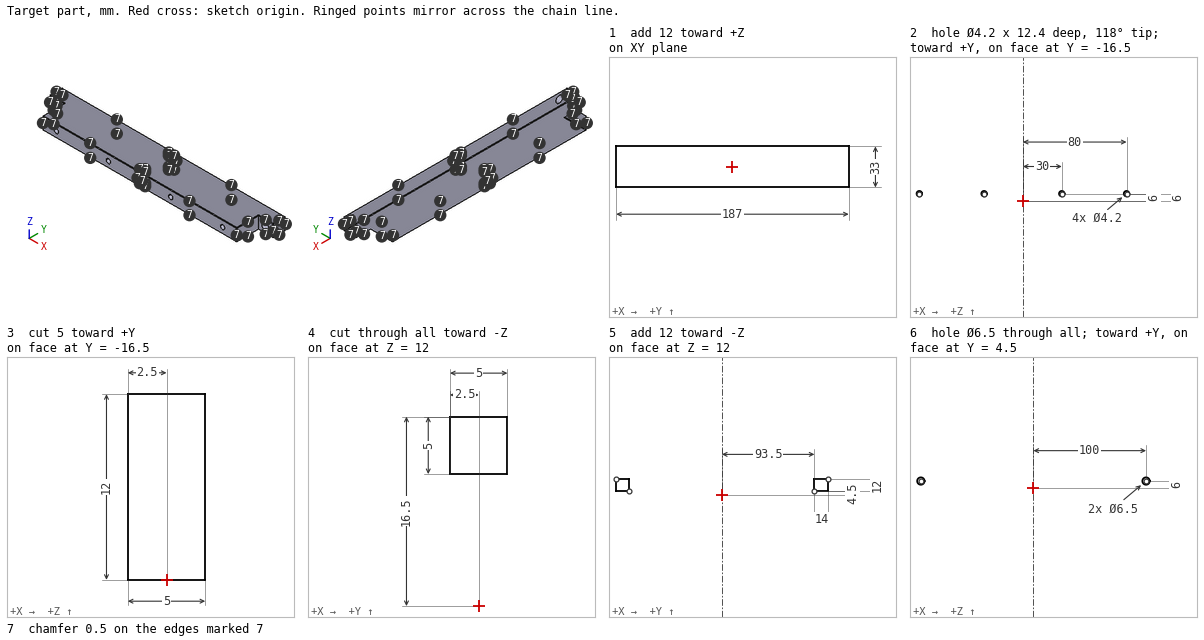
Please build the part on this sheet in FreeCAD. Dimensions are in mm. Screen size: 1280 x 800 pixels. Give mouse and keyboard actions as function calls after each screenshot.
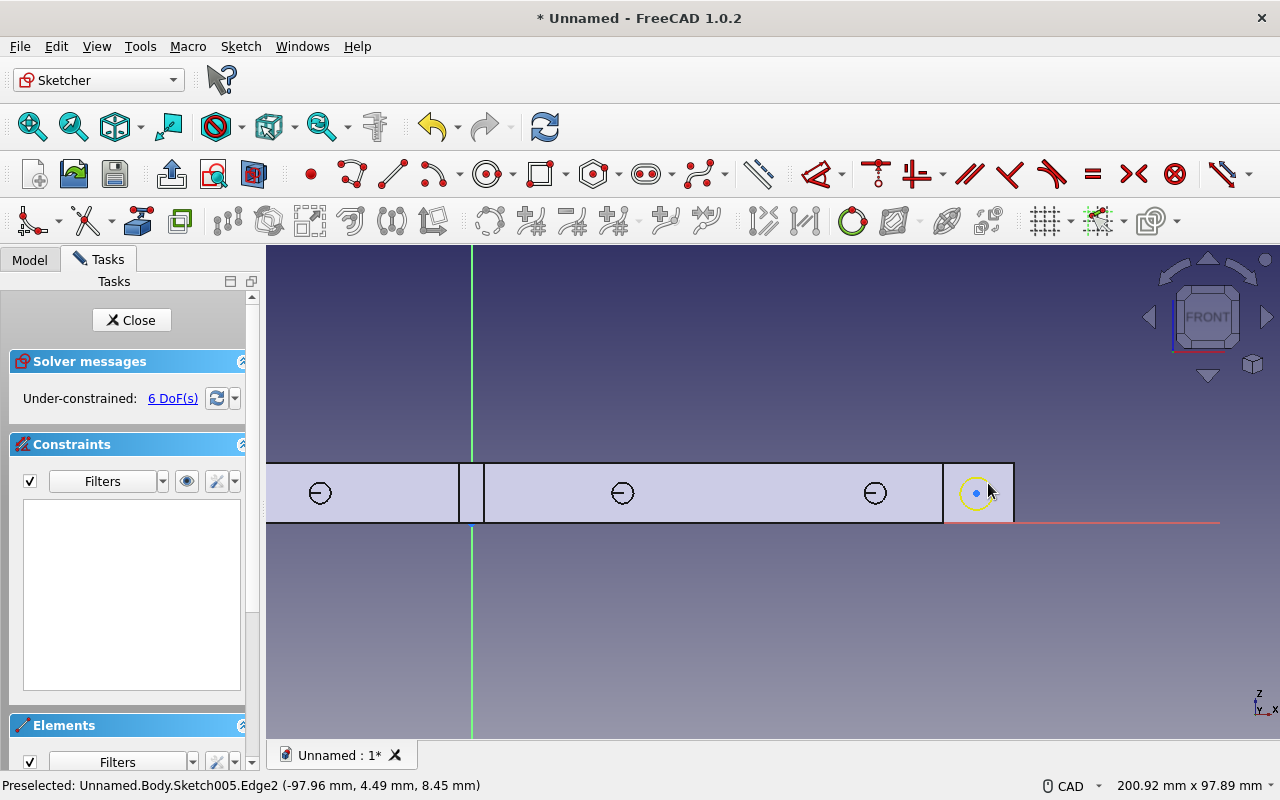
click(988, 482)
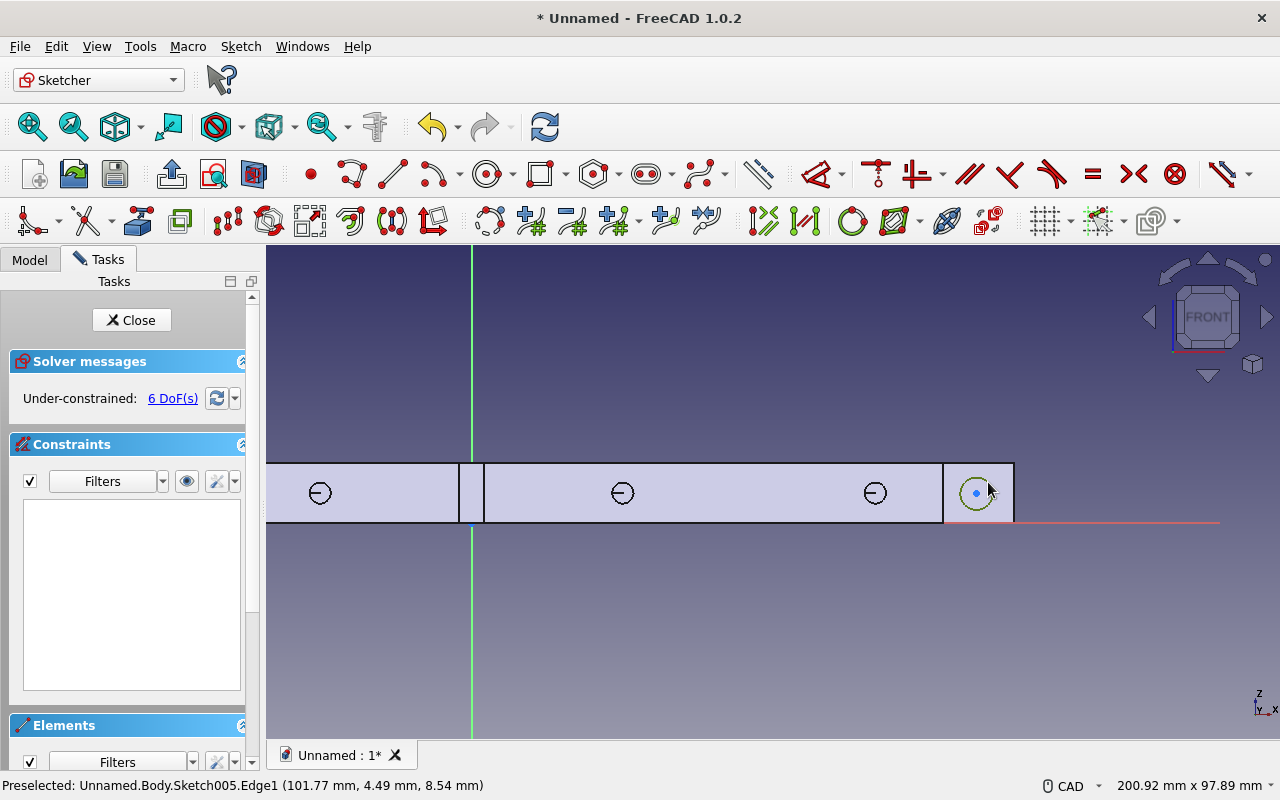
scroll(988, 482, down, 3)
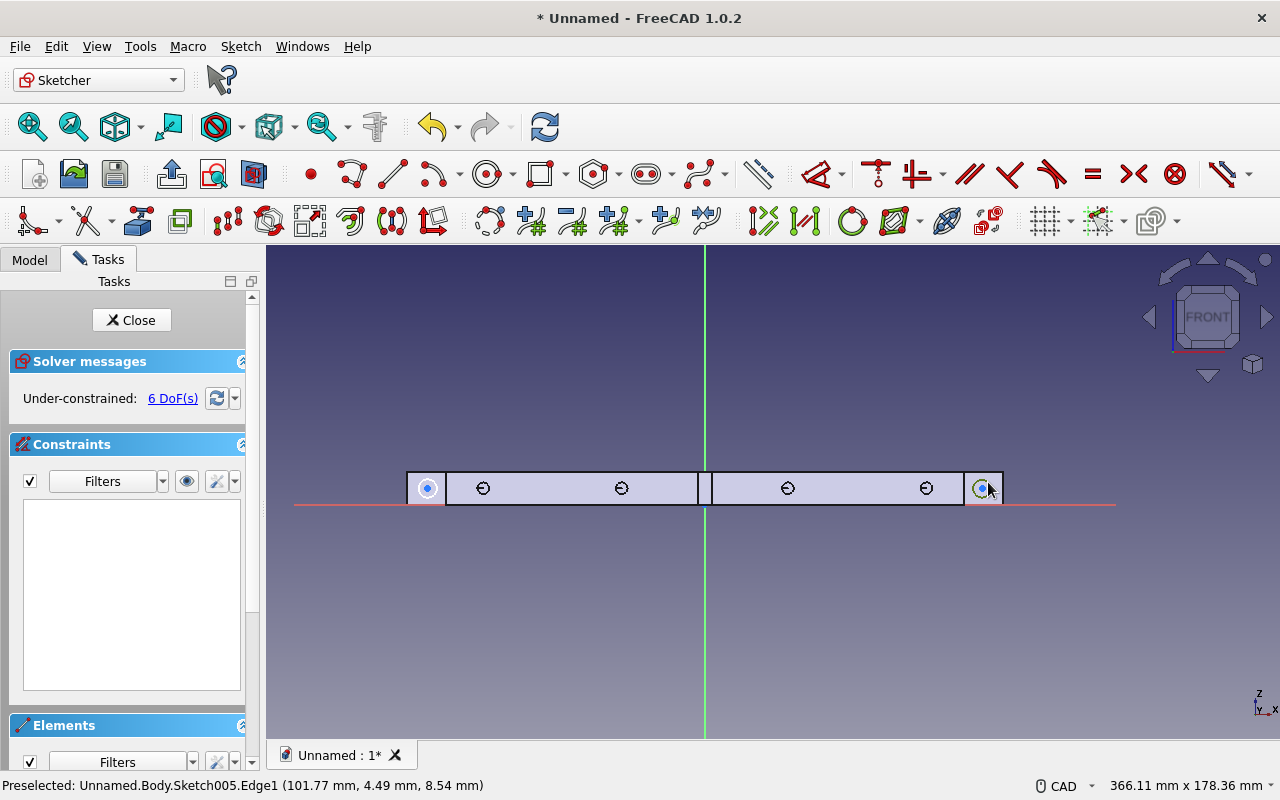
scroll(434, 482, up, 3)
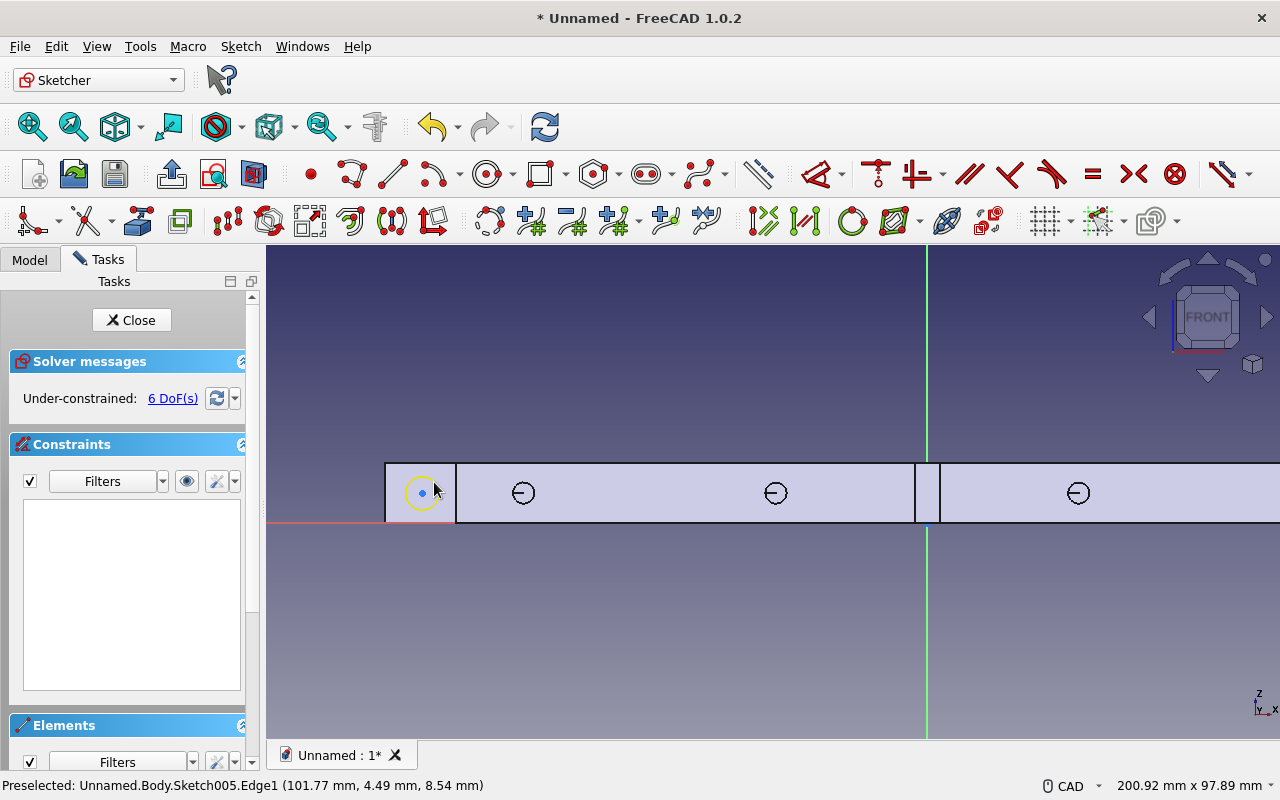
click(434, 482)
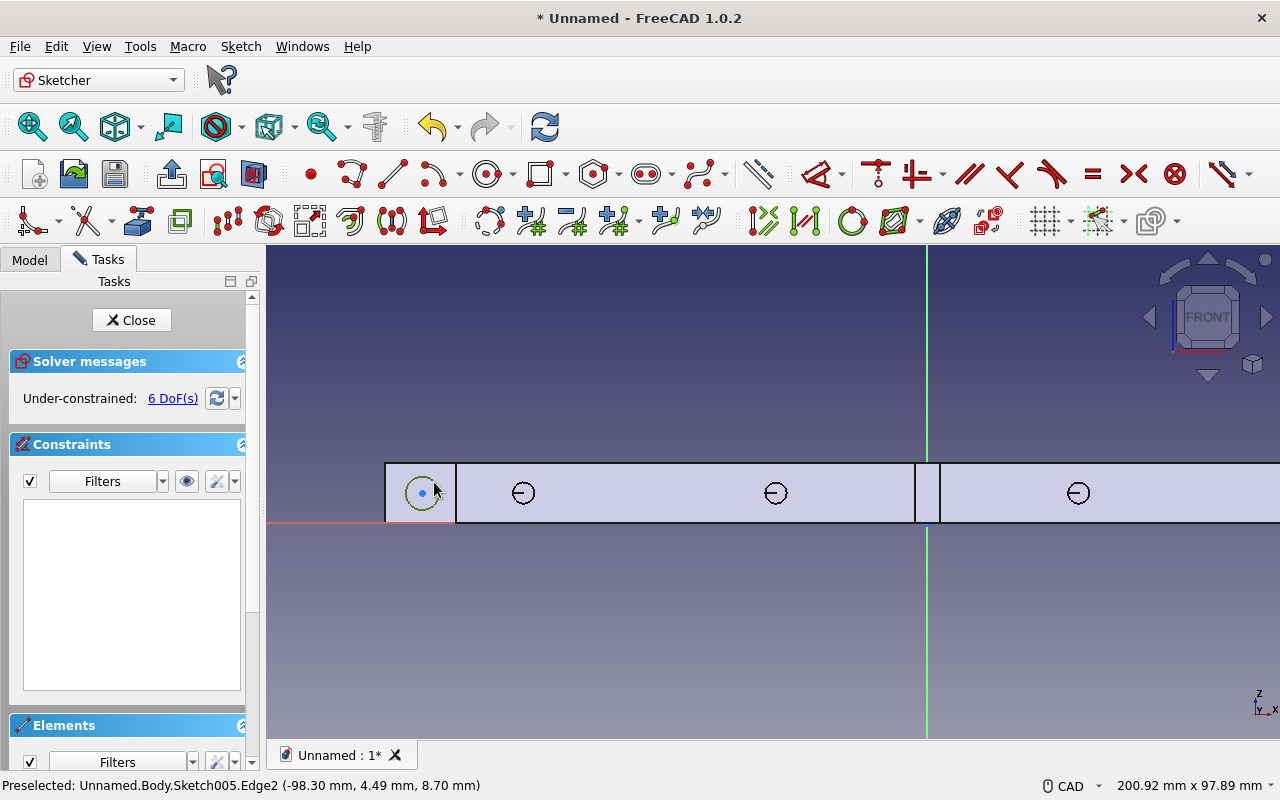
key(e)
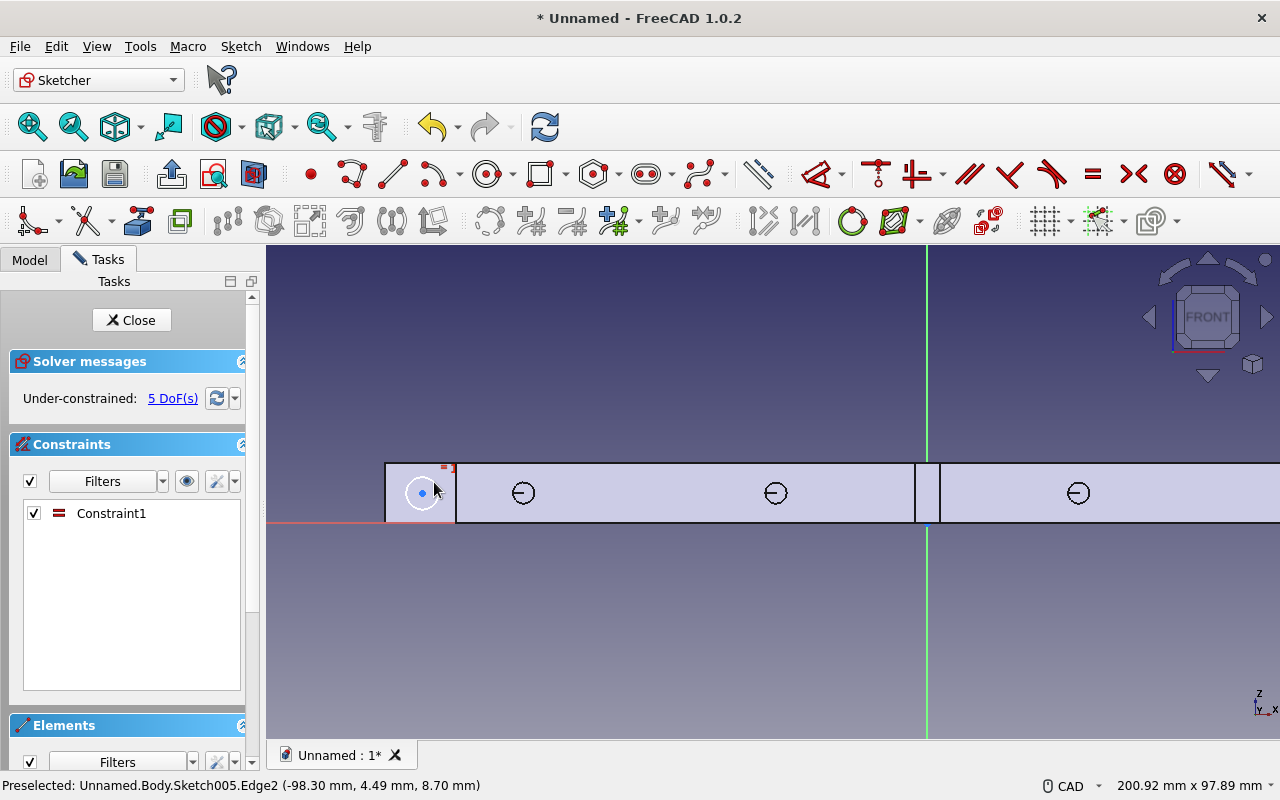
scroll(433, 482, down, 3)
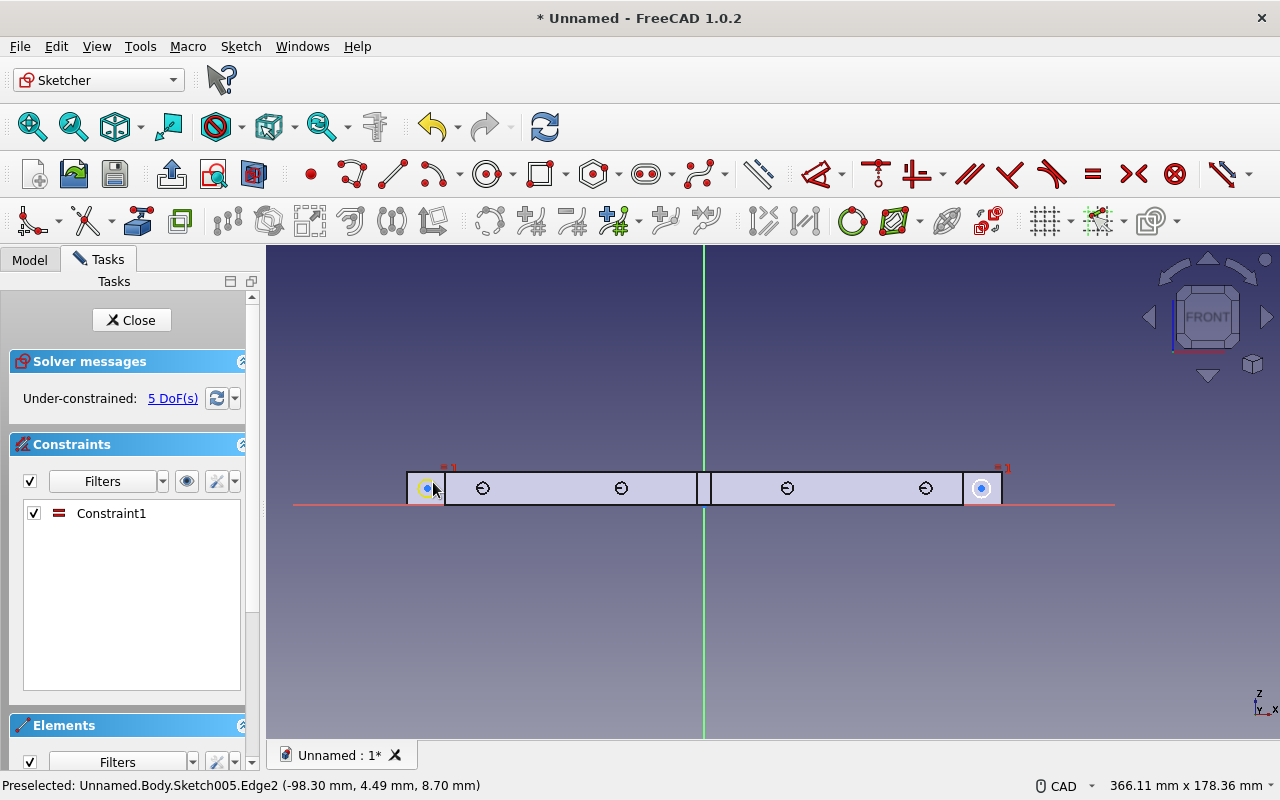
click(982, 489)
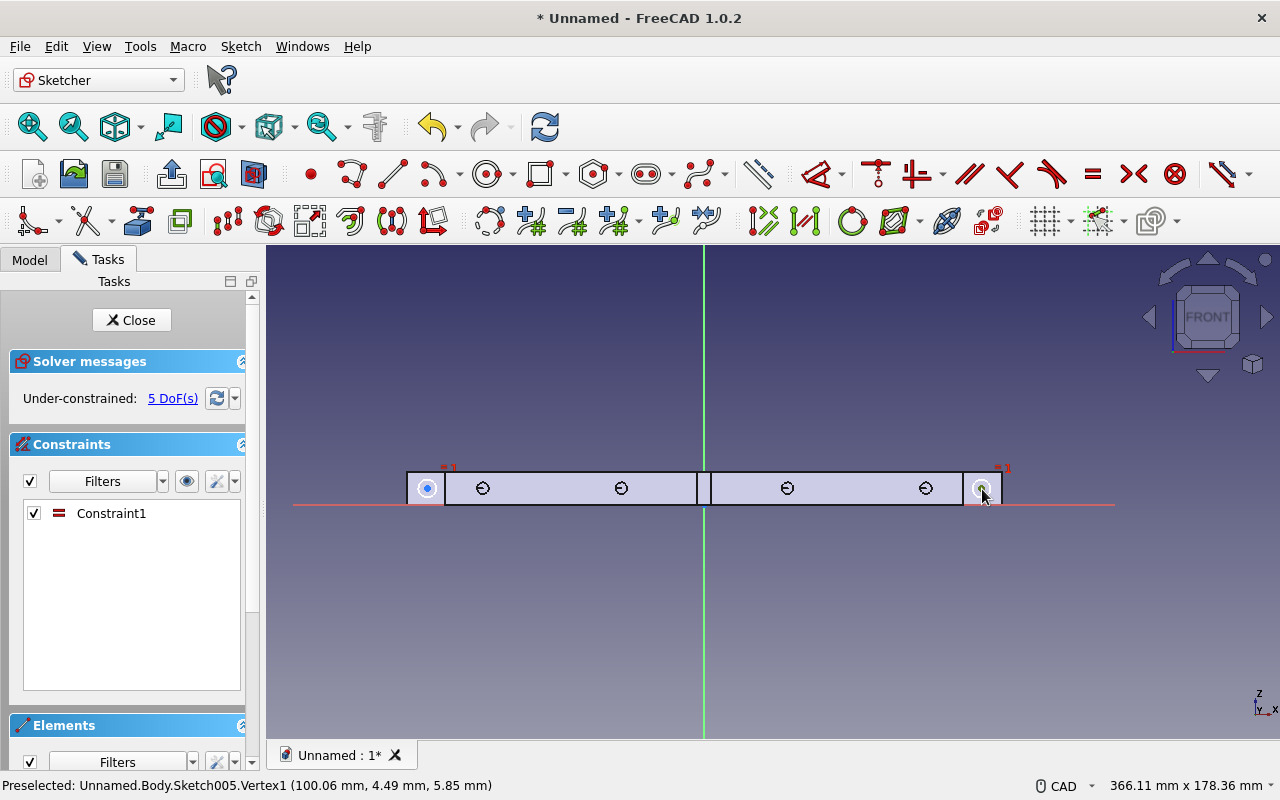
click(427, 488)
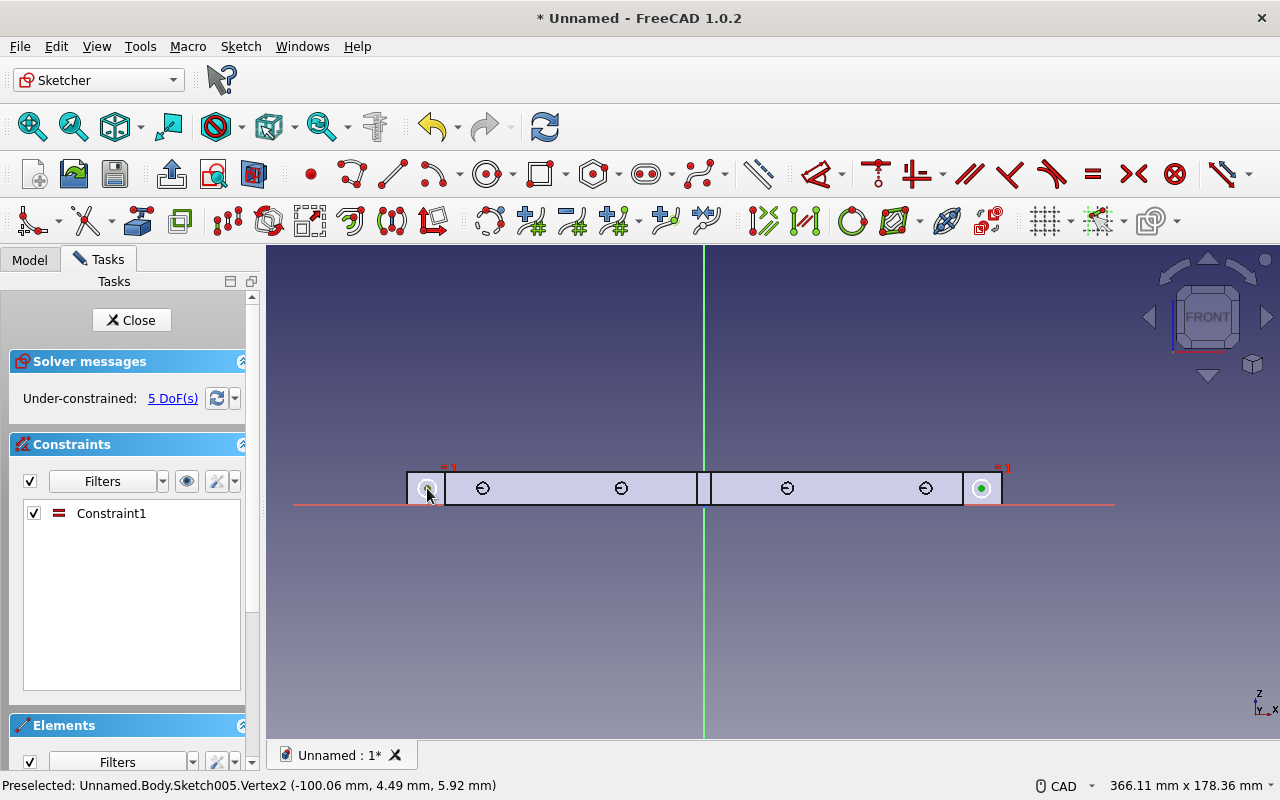
click(704, 680)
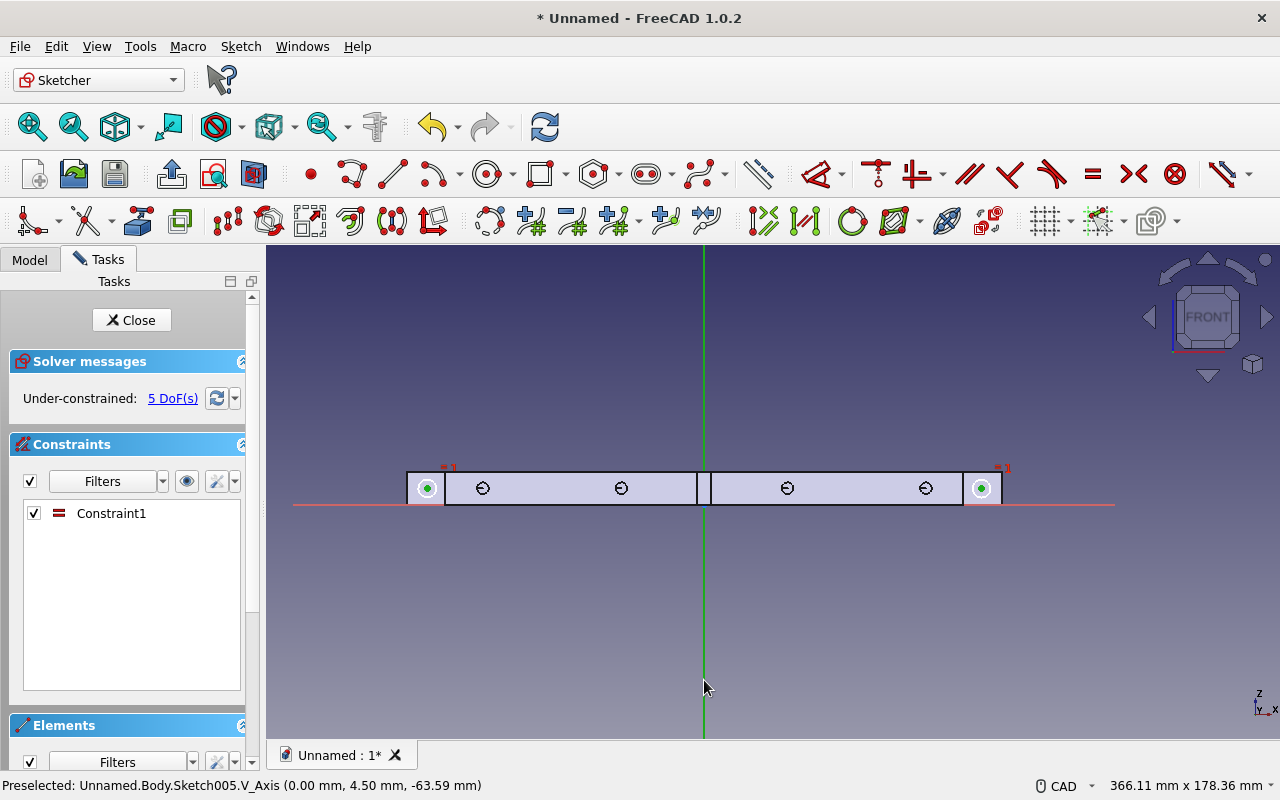
key(s)